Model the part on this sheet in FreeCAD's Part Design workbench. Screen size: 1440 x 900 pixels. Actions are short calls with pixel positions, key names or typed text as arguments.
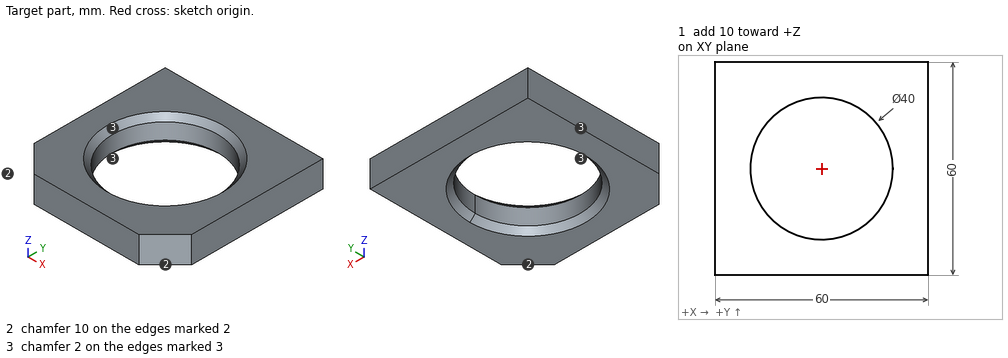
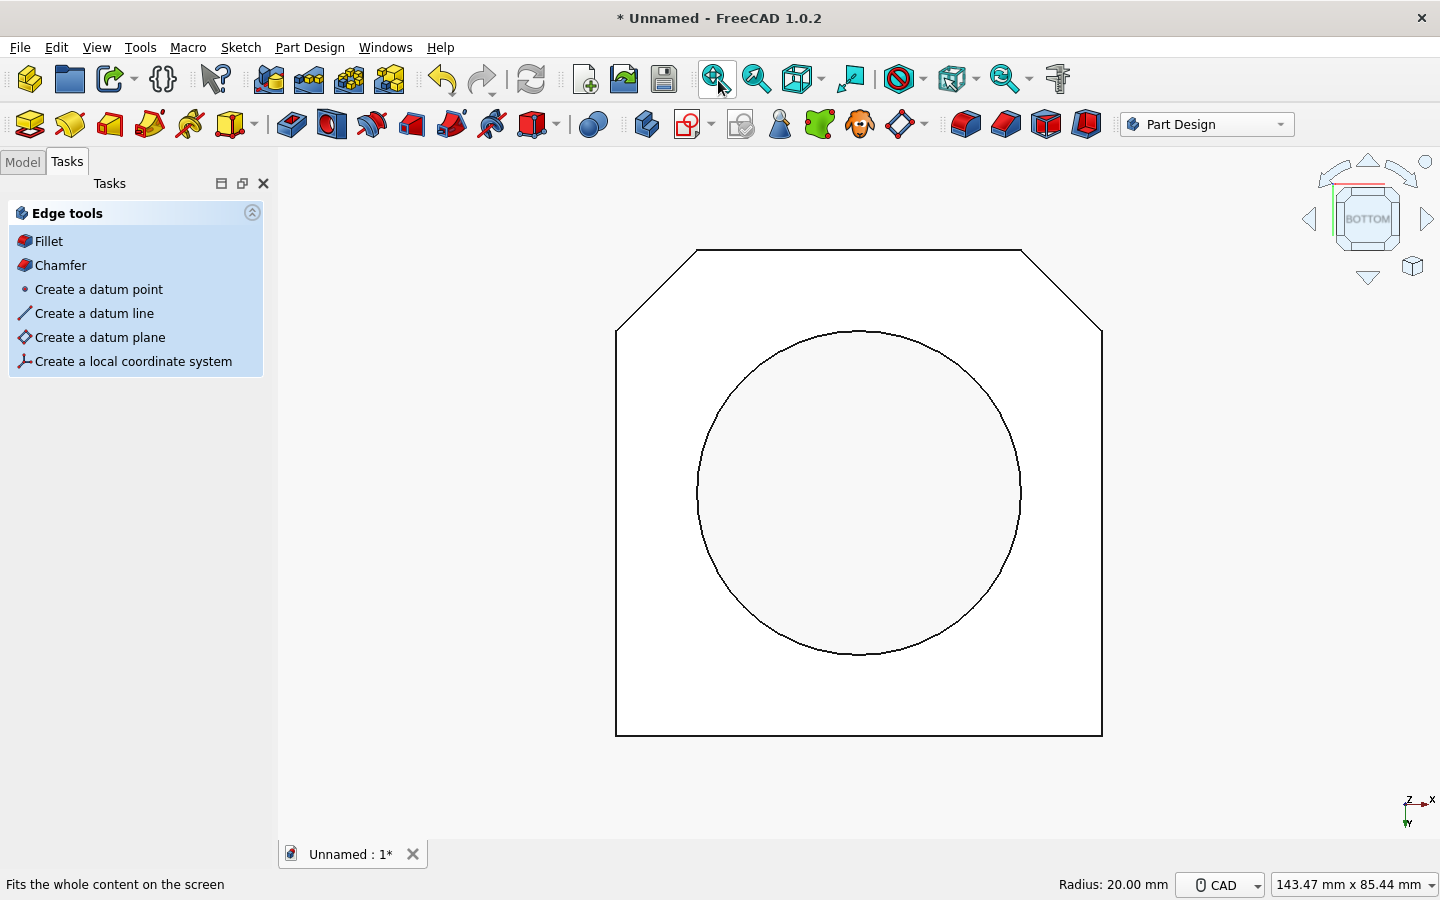
click(697, 492, ctrl)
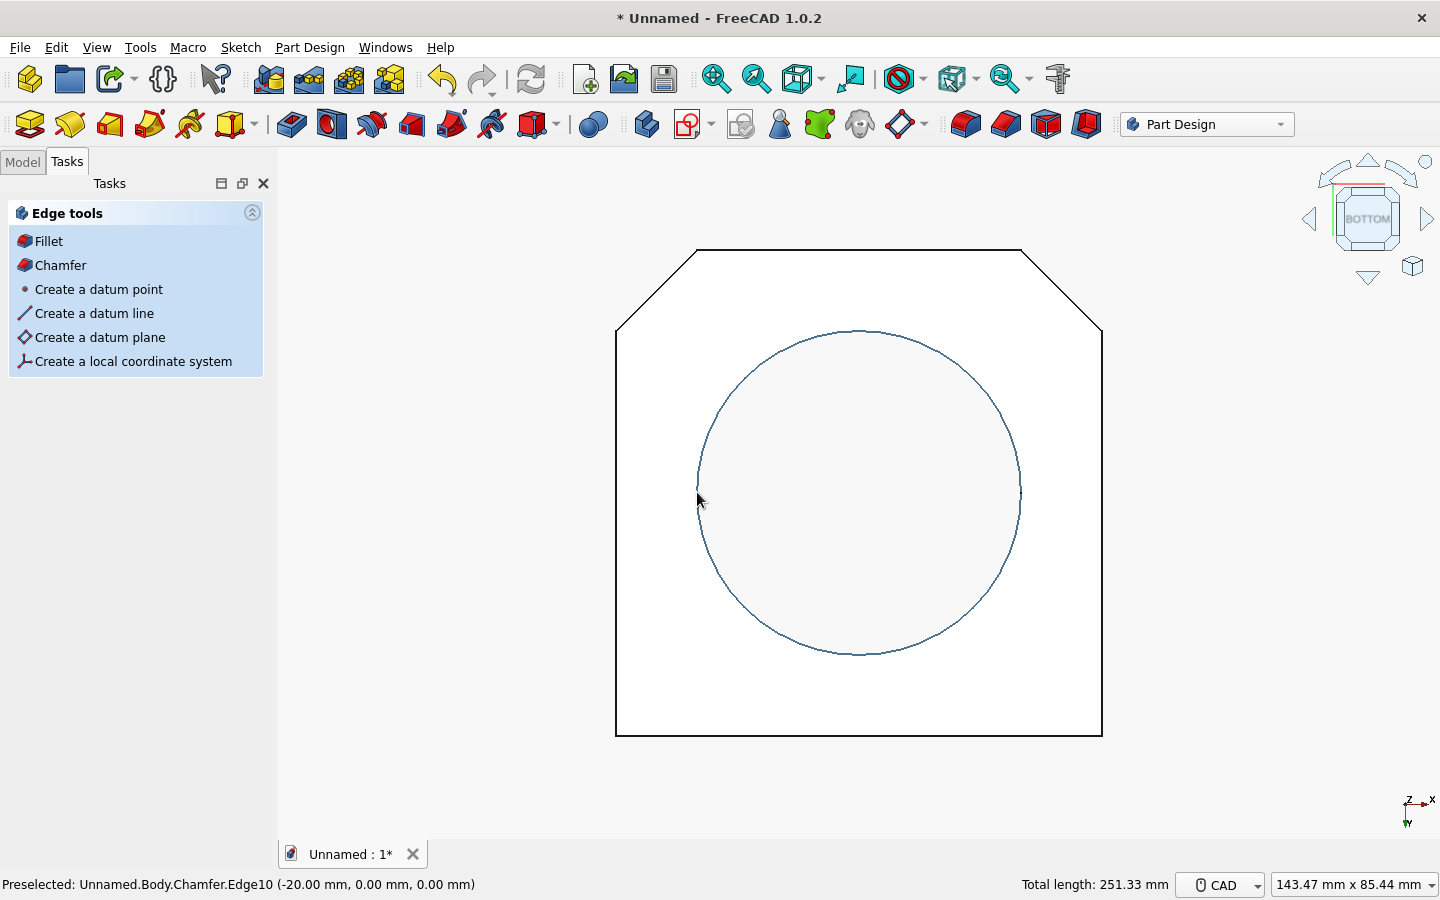
click(1006, 124)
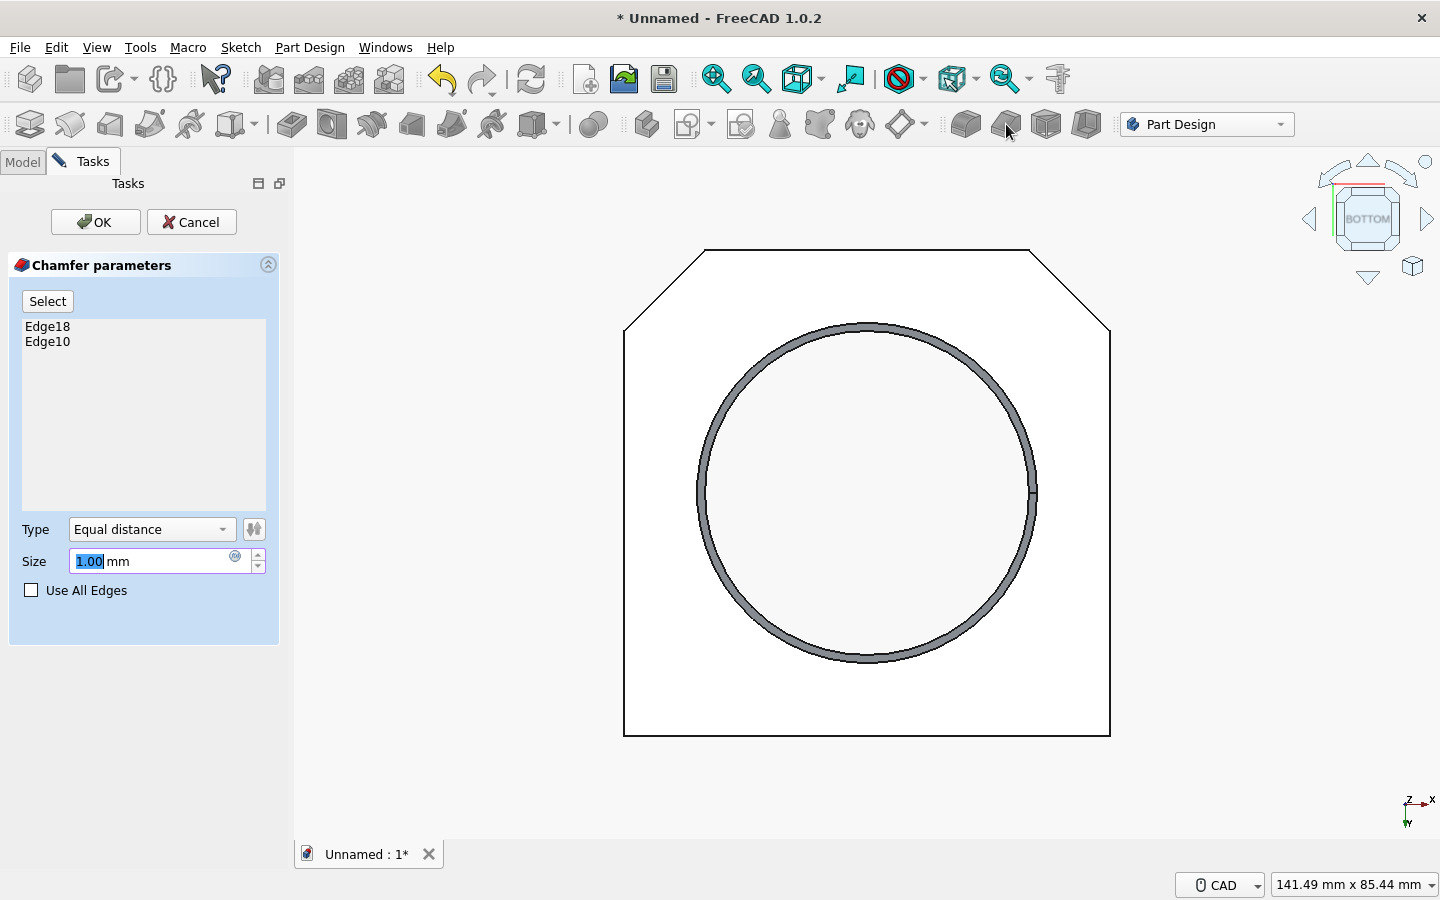
text(2)
key(Tab)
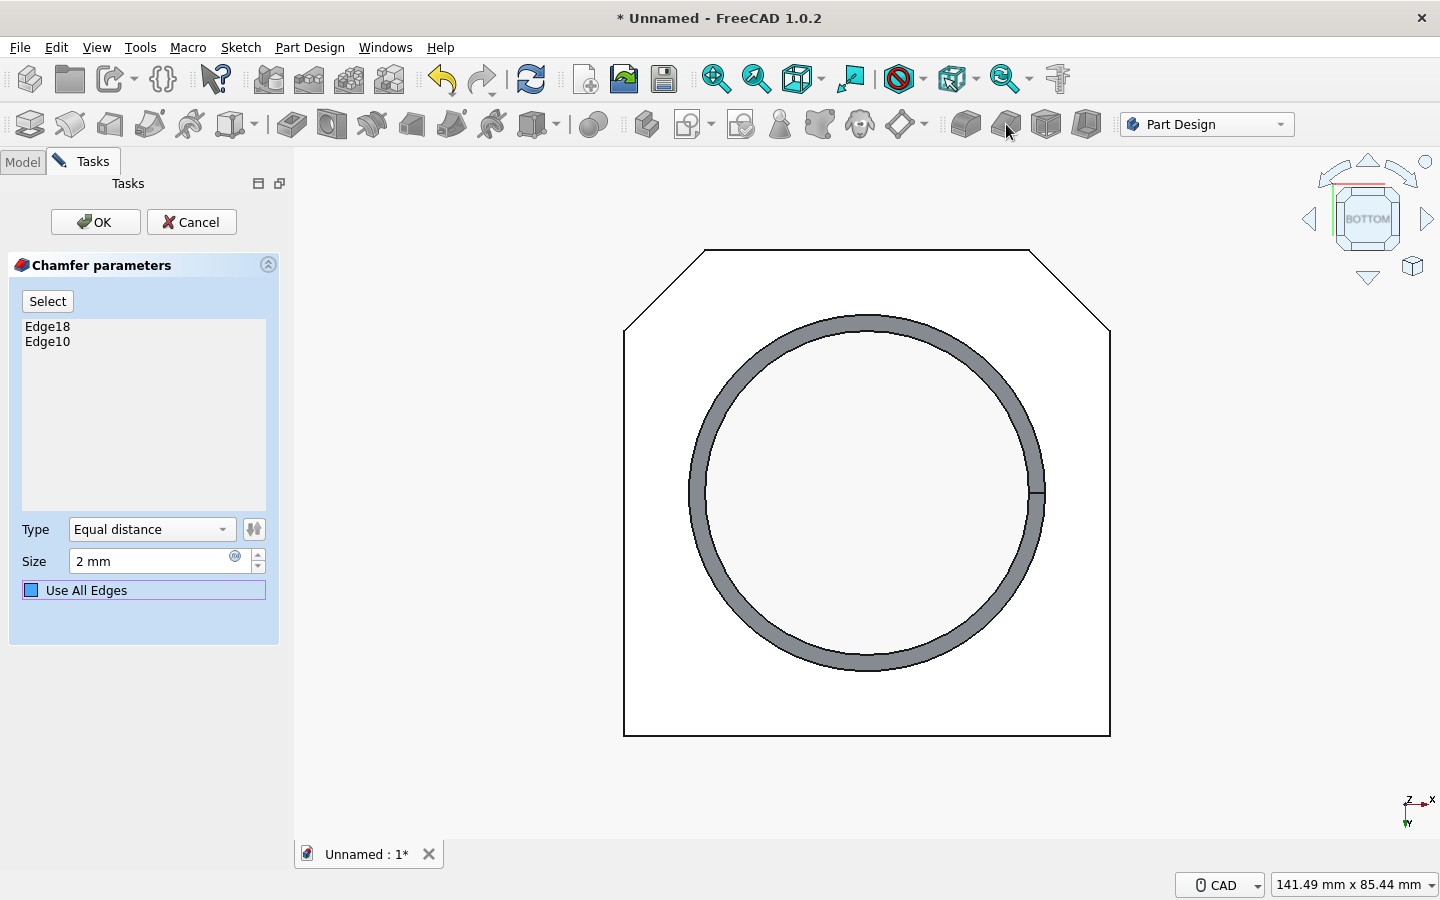
click(96, 222)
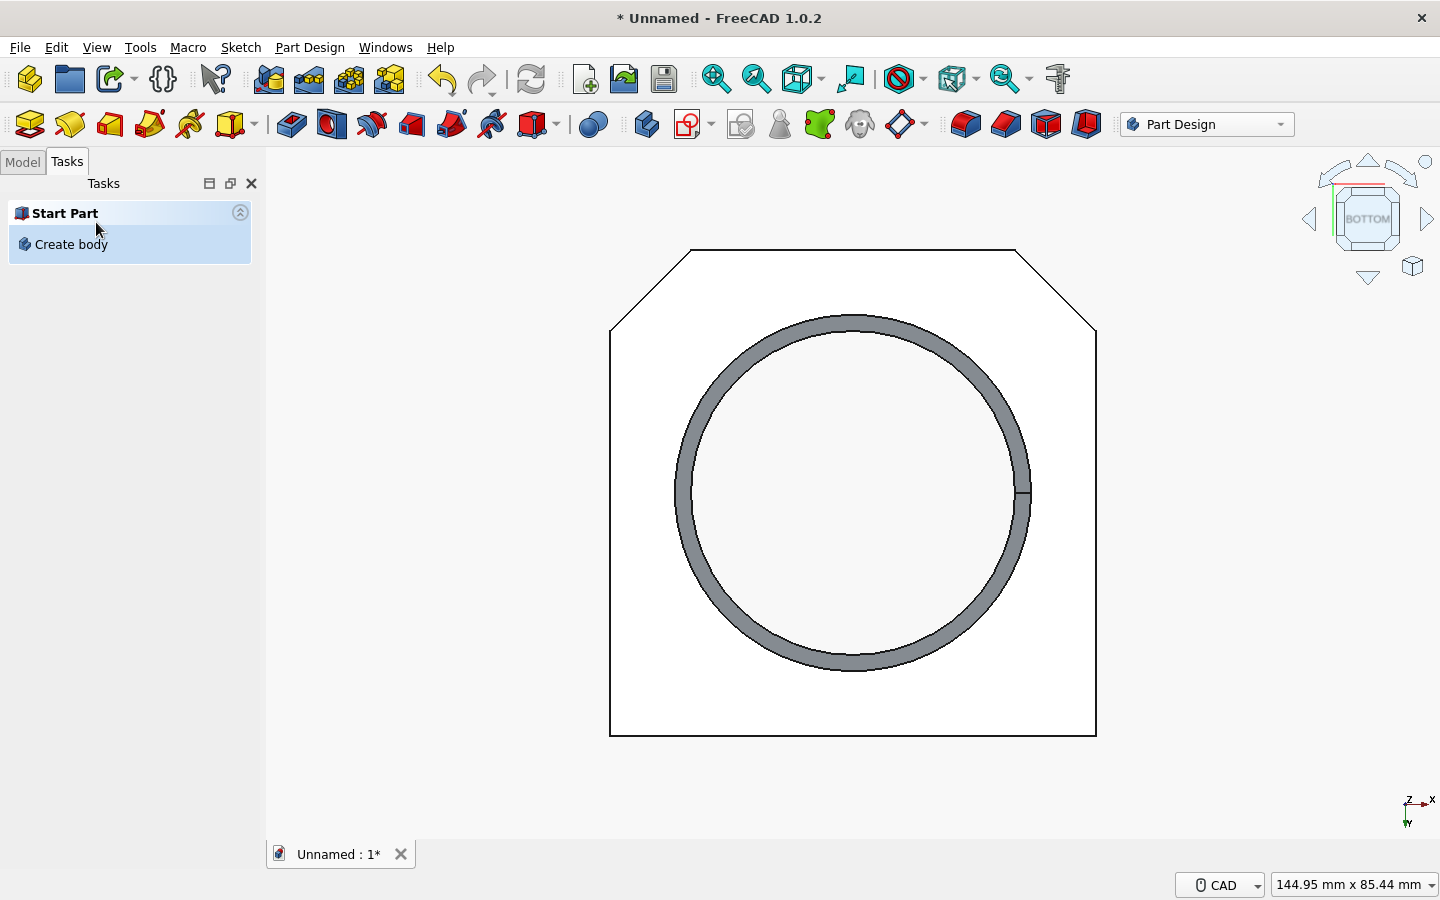
key(0)